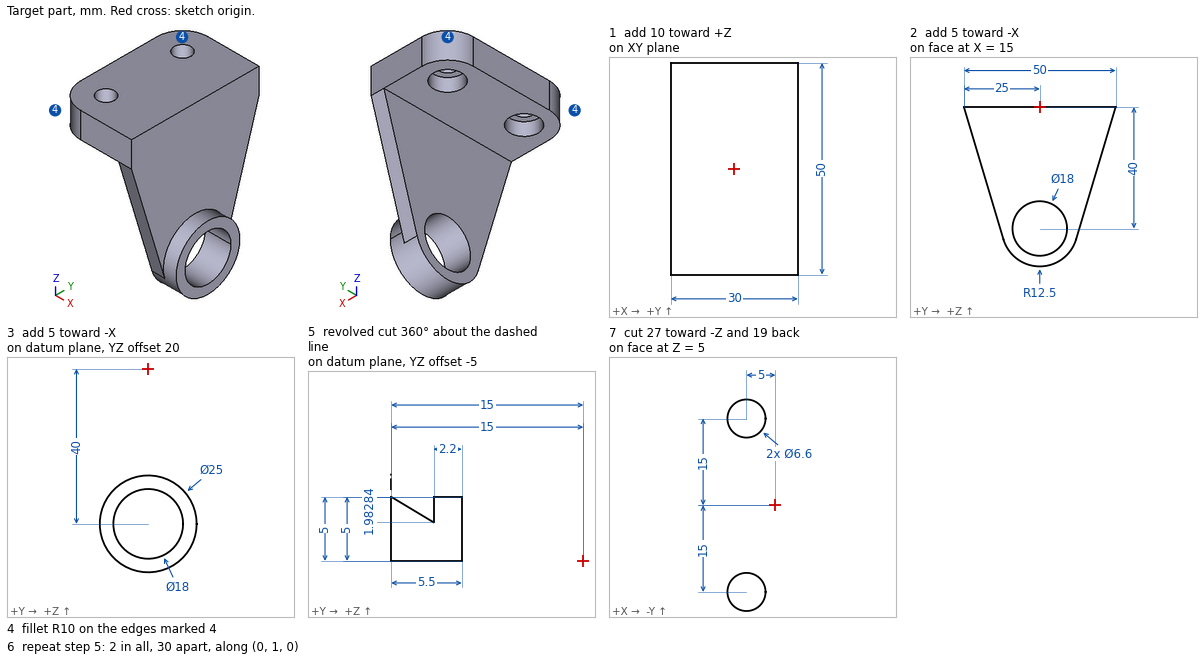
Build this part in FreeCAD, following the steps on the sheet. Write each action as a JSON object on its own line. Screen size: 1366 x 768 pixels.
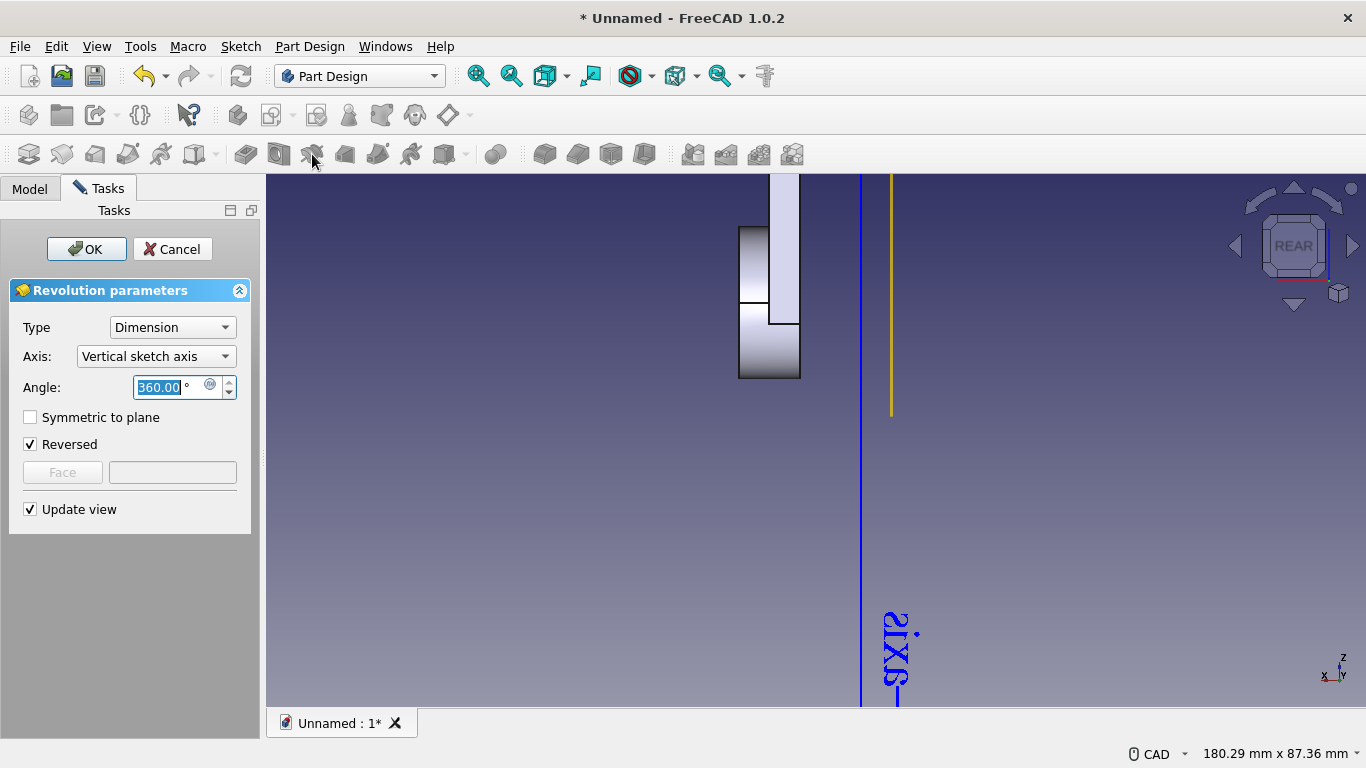
{"action": "left_click", "coordinate": [157, 356]}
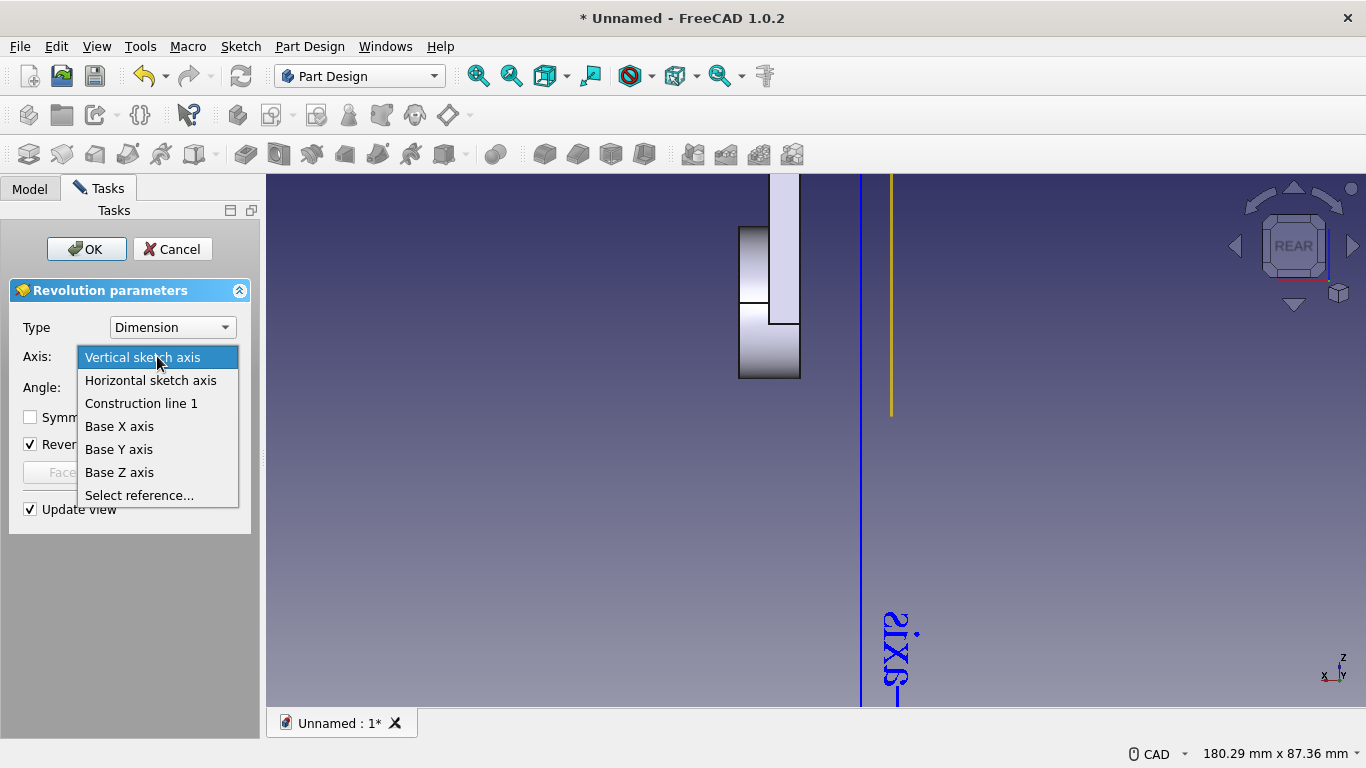
{"action": "left_click", "coordinate": [156, 404]}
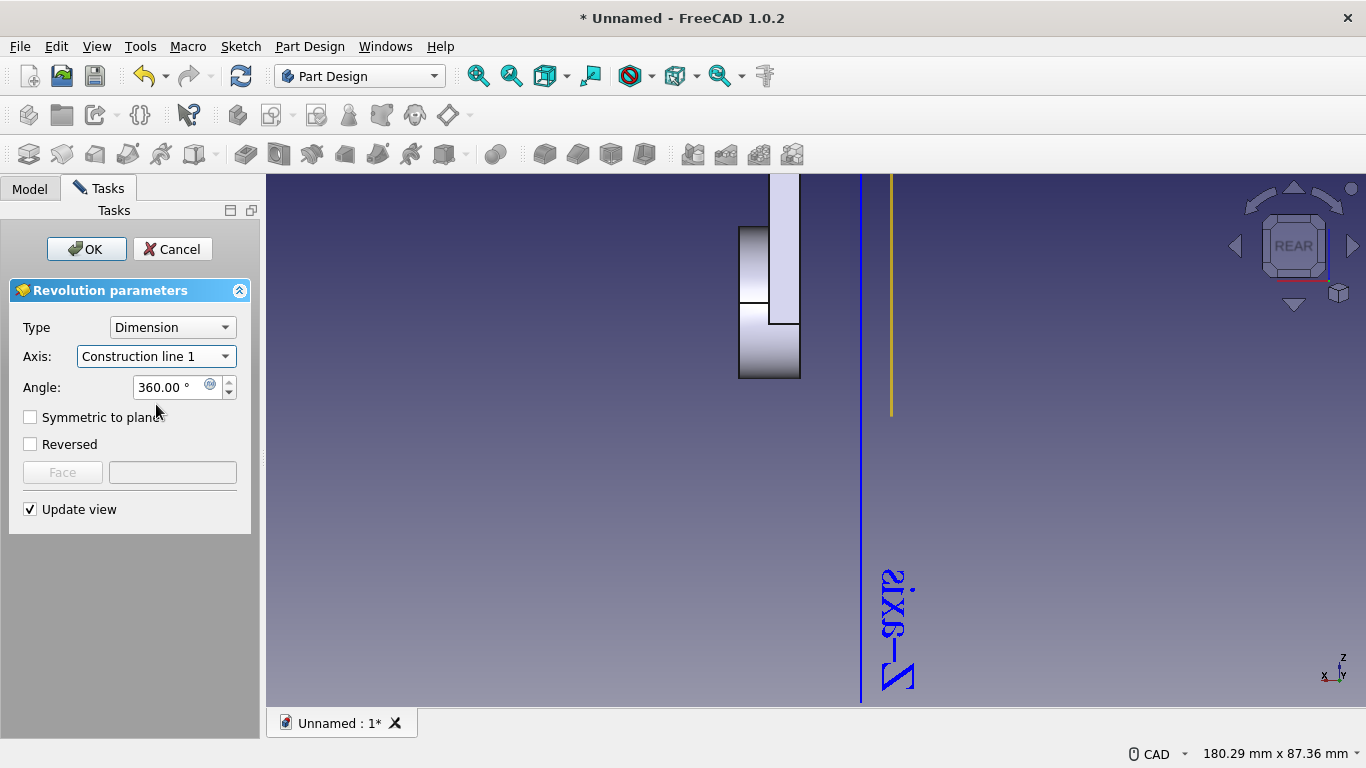
{"action": "left_click", "coordinate": [87, 249]}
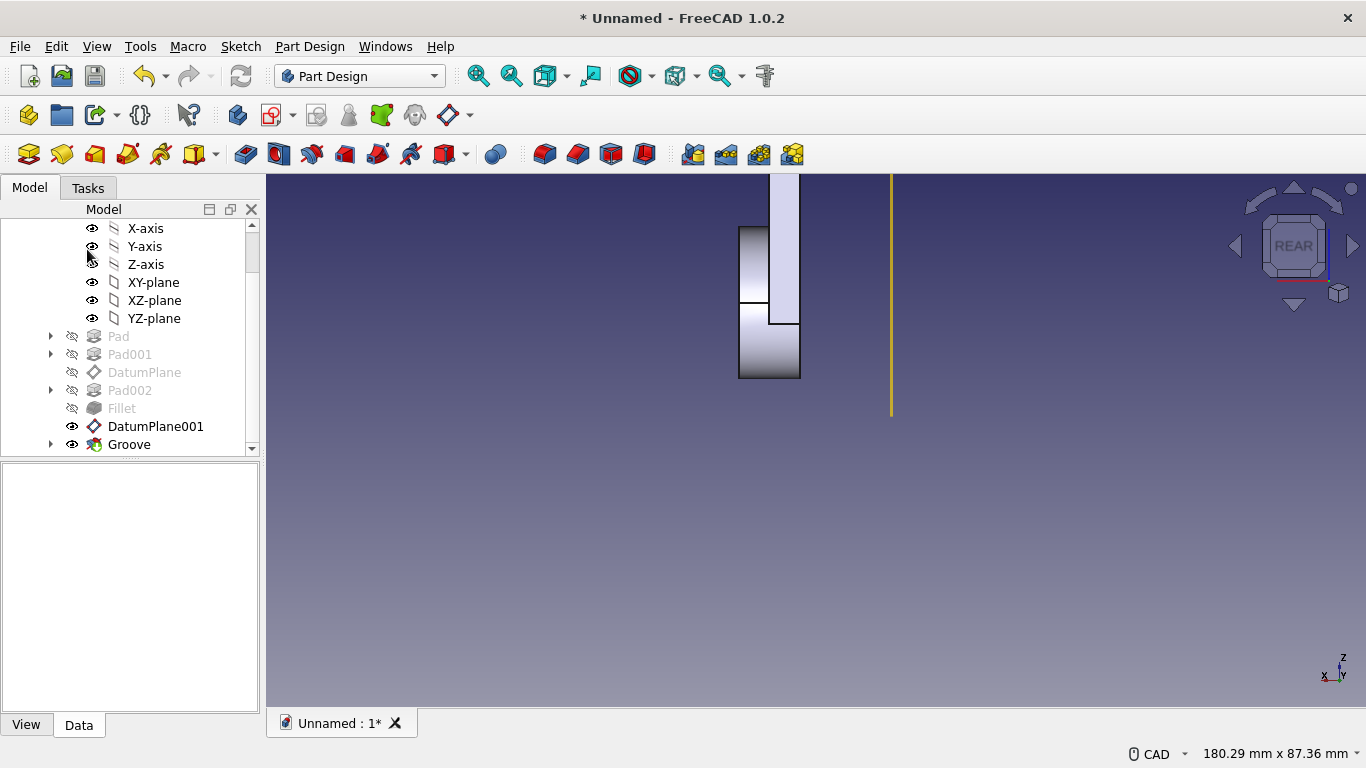
{"action": "left_click", "coordinate": [117, 426]}
{"action": "key", "text": "space"}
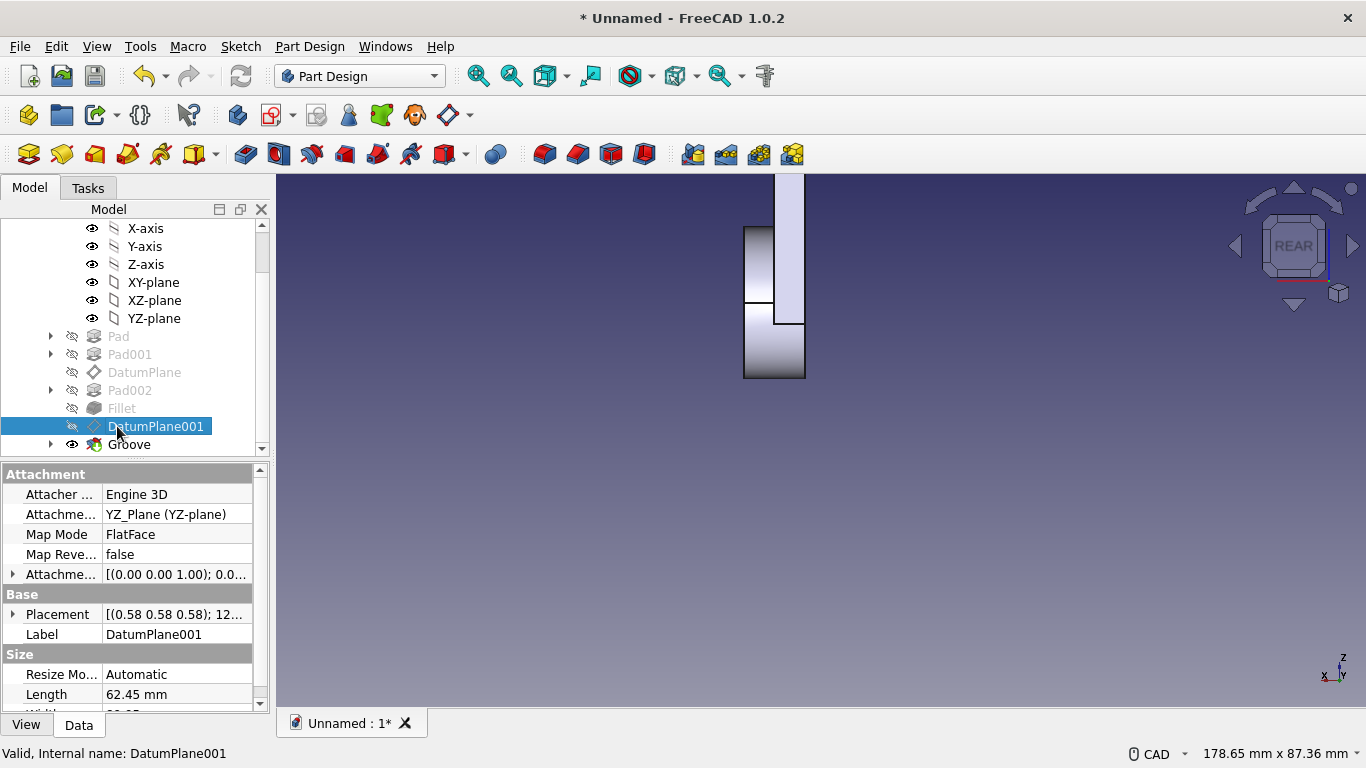
{"action": "left_click", "coordinate": [479, 76]}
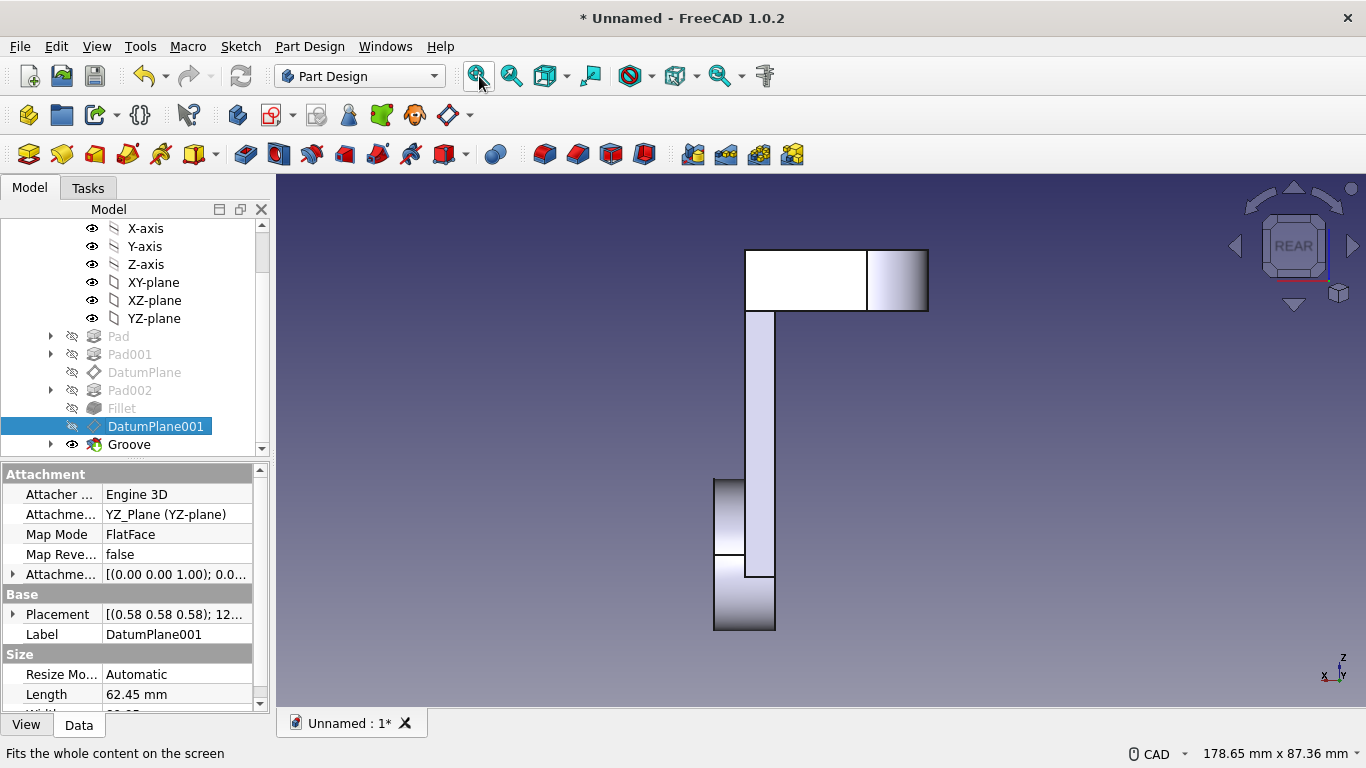
{"action": "left_click", "coordinate": [117, 444]}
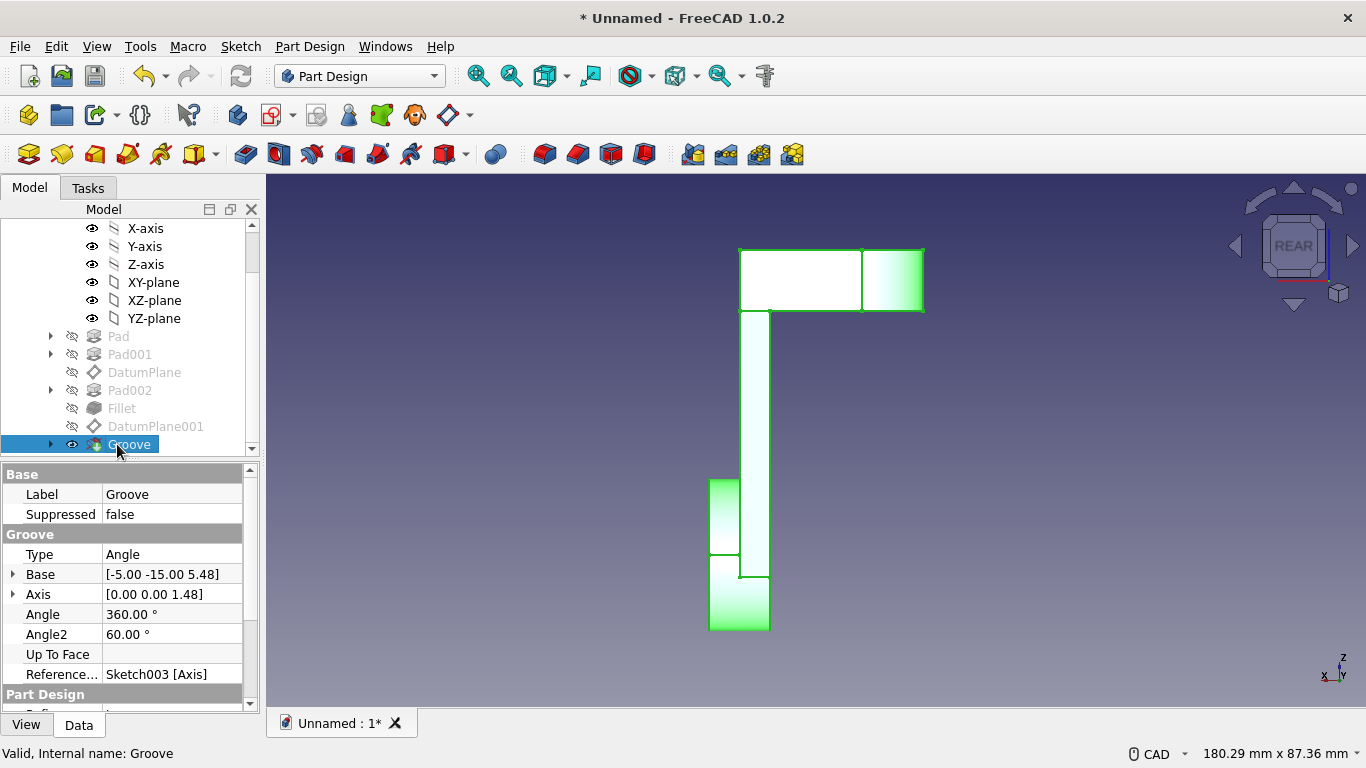
{"action": "left_click", "coordinate": [726, 154]}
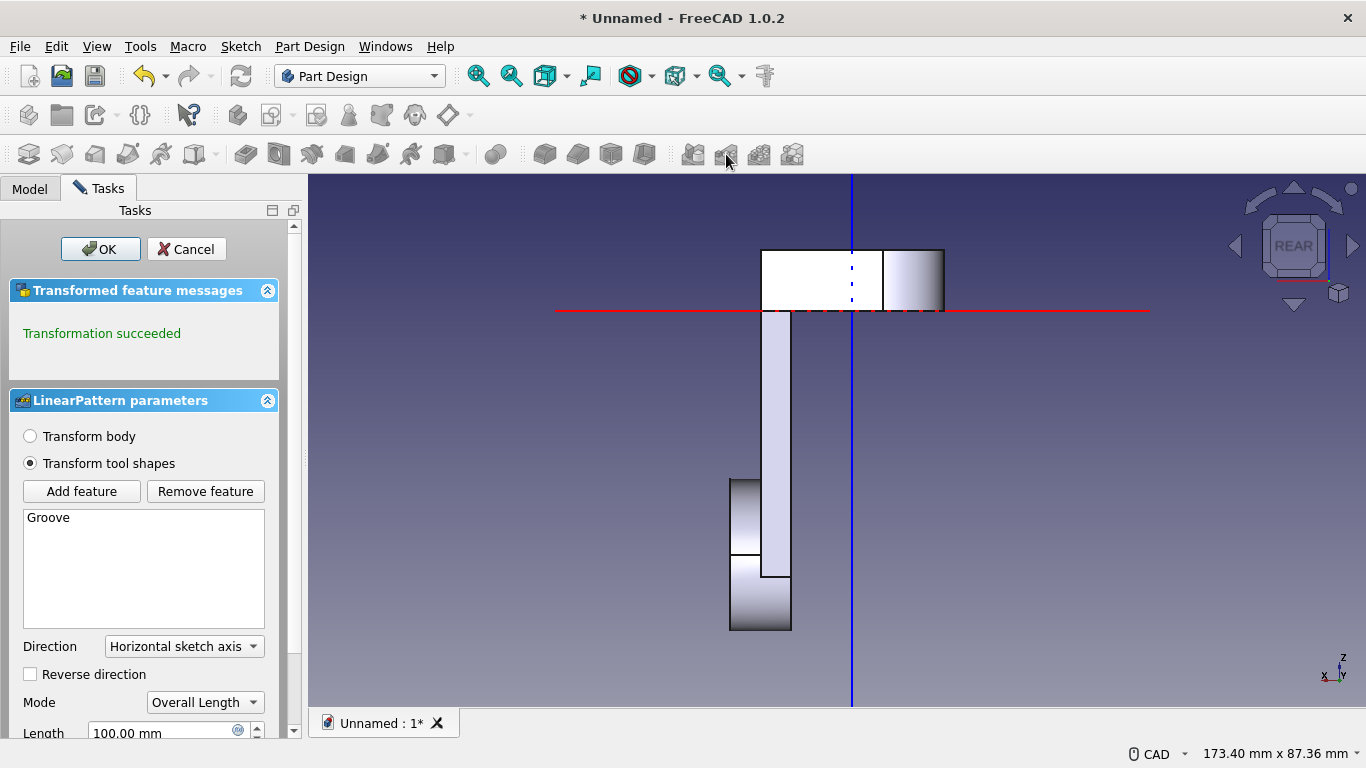
{"action": "left_click", "coordinate": [185, 646]}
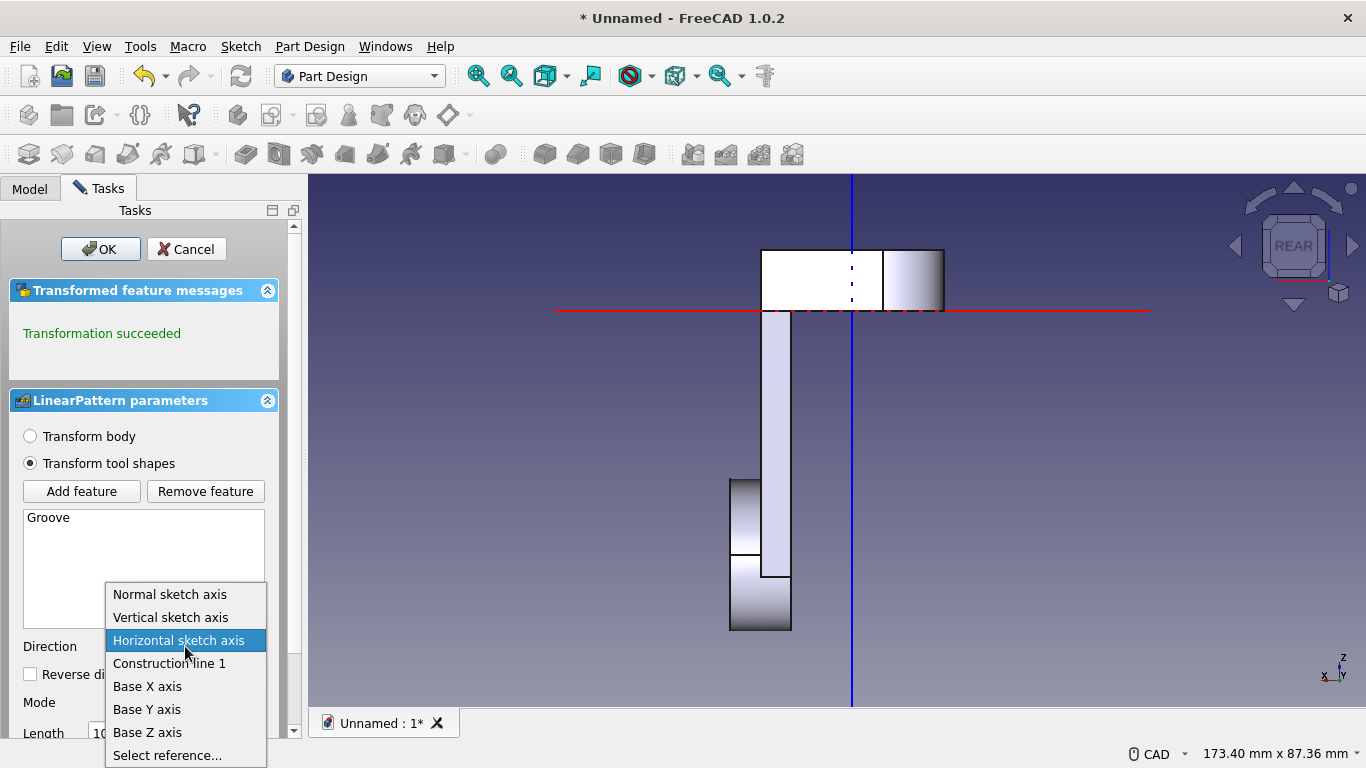
{"action": "left_click", "coordinate": [184, 710]}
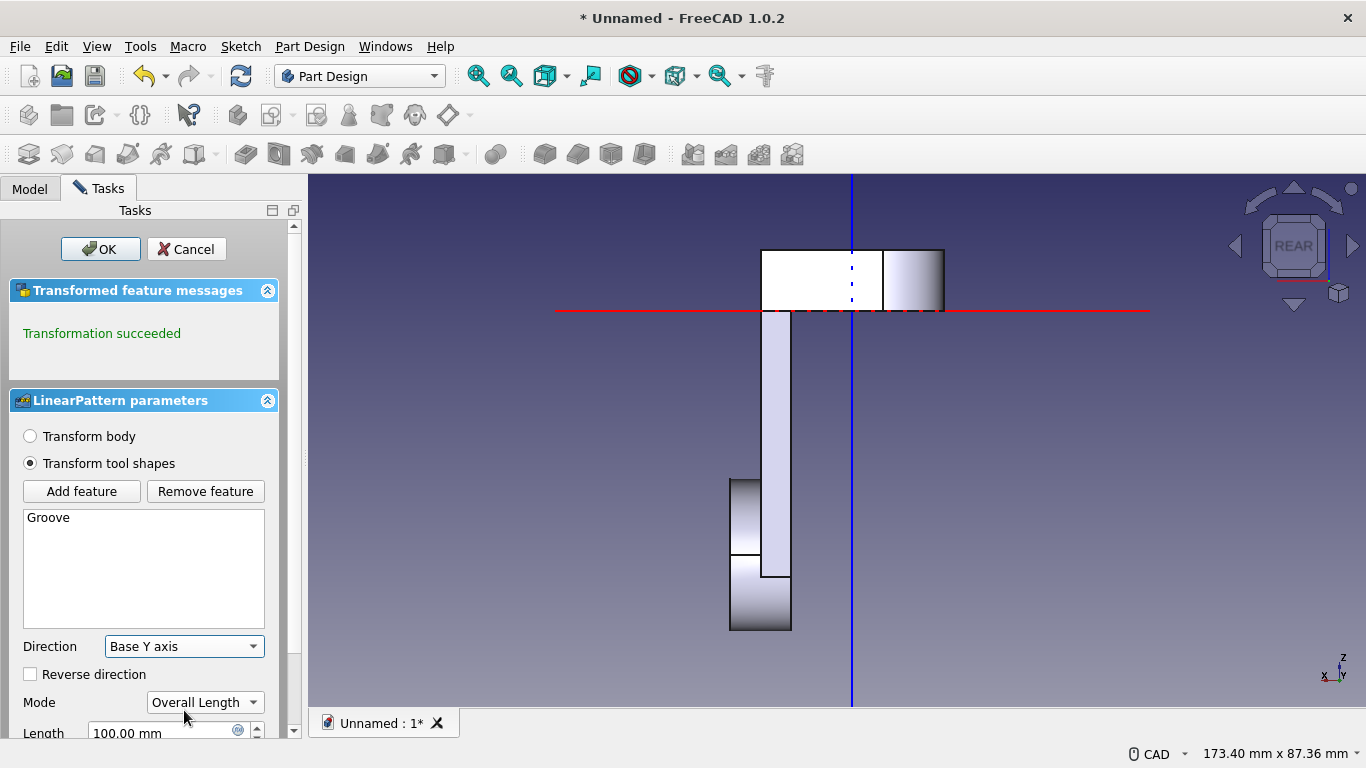
{"action": "left_click", "coordinate": [206, 702]}